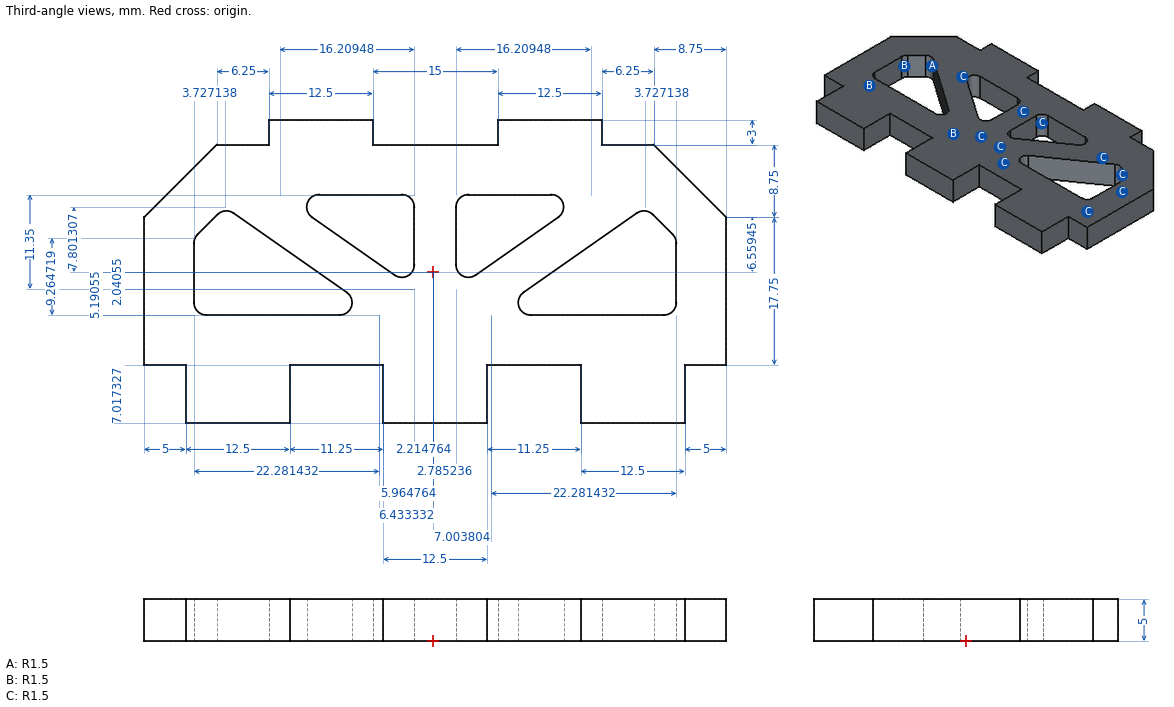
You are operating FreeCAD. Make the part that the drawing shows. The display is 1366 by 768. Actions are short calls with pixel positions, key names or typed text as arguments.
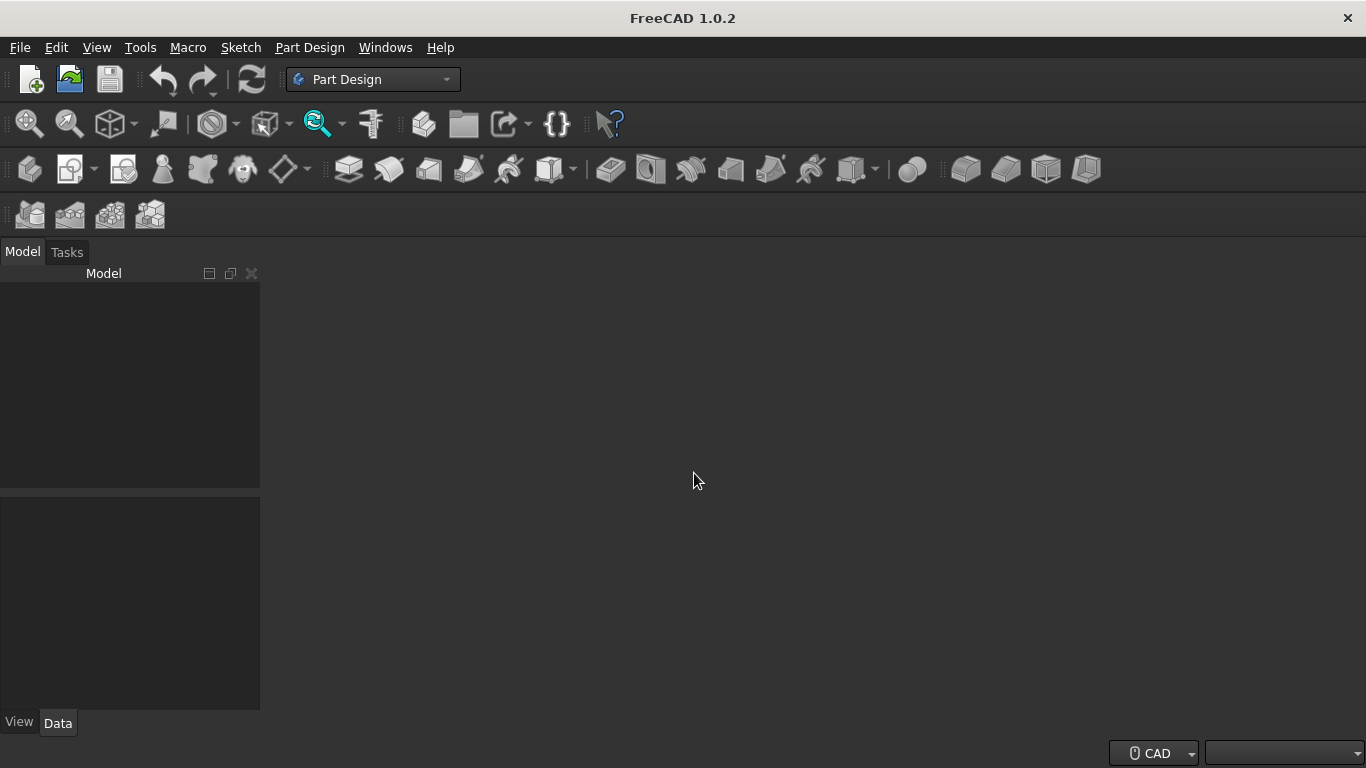
key(ctrl+n)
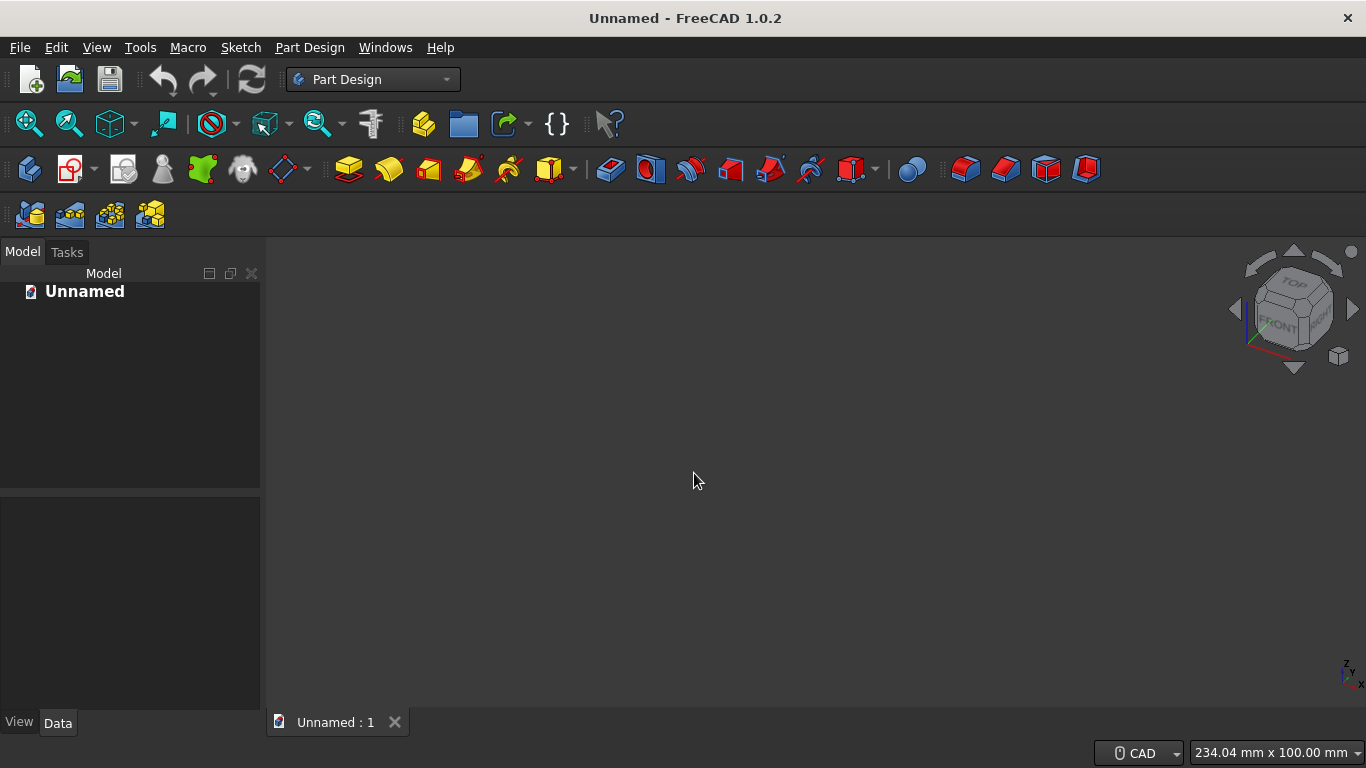
click(70, 170)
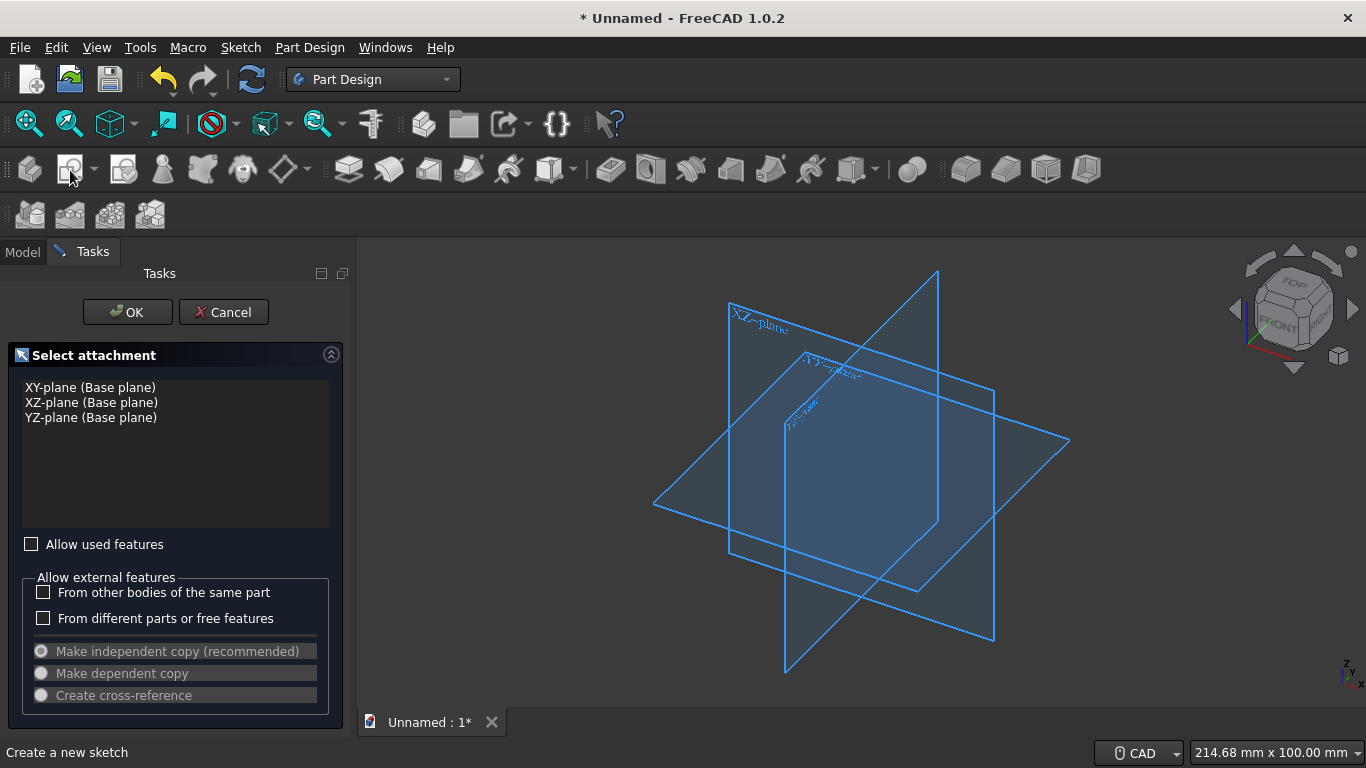
click(82, 388)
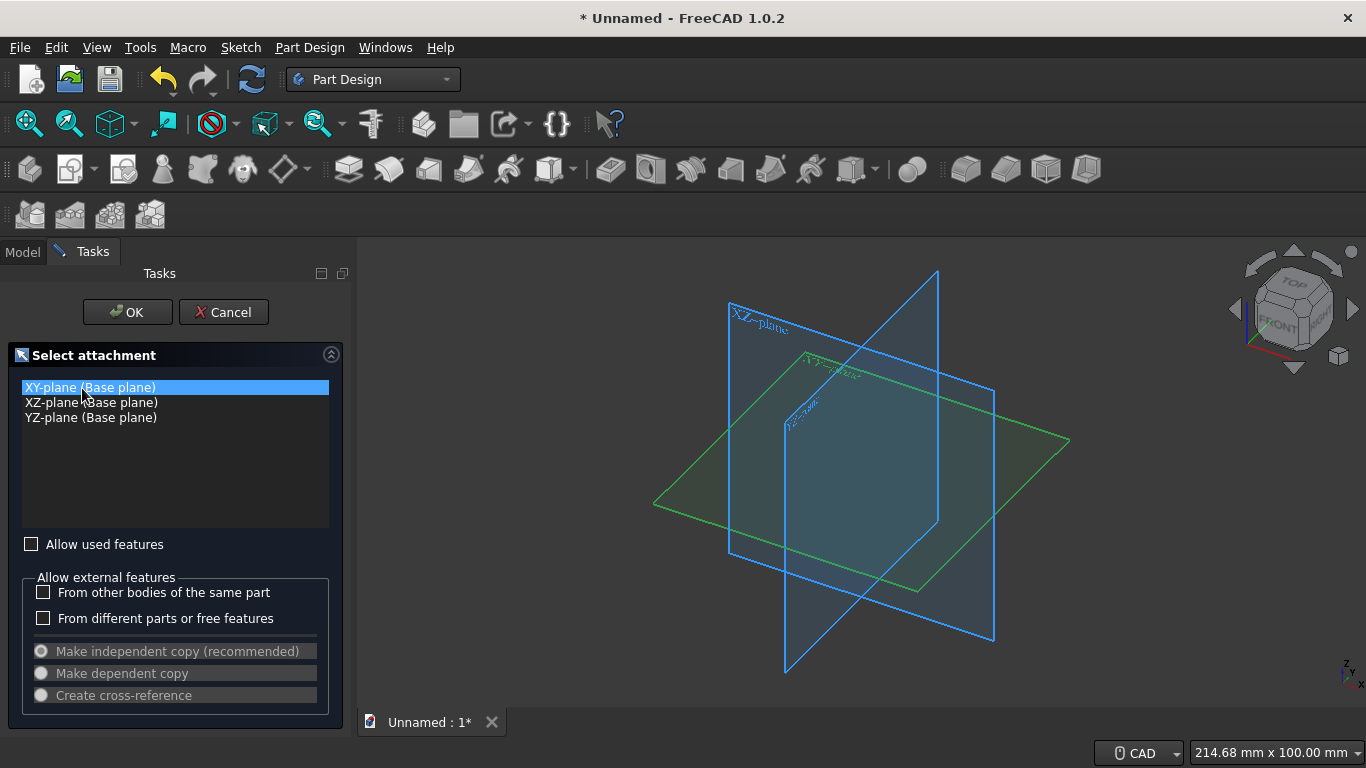
click(128, 312)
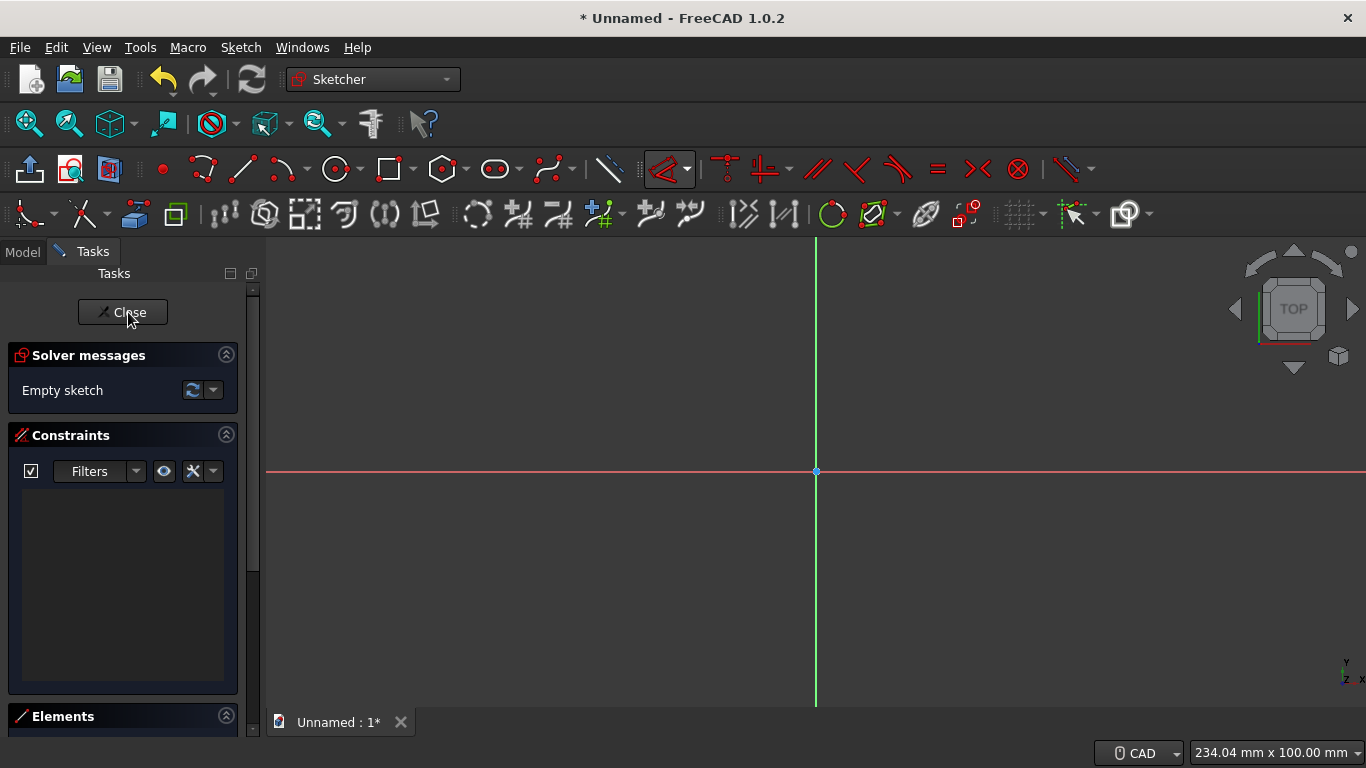
scroll(902, 471, up, 3)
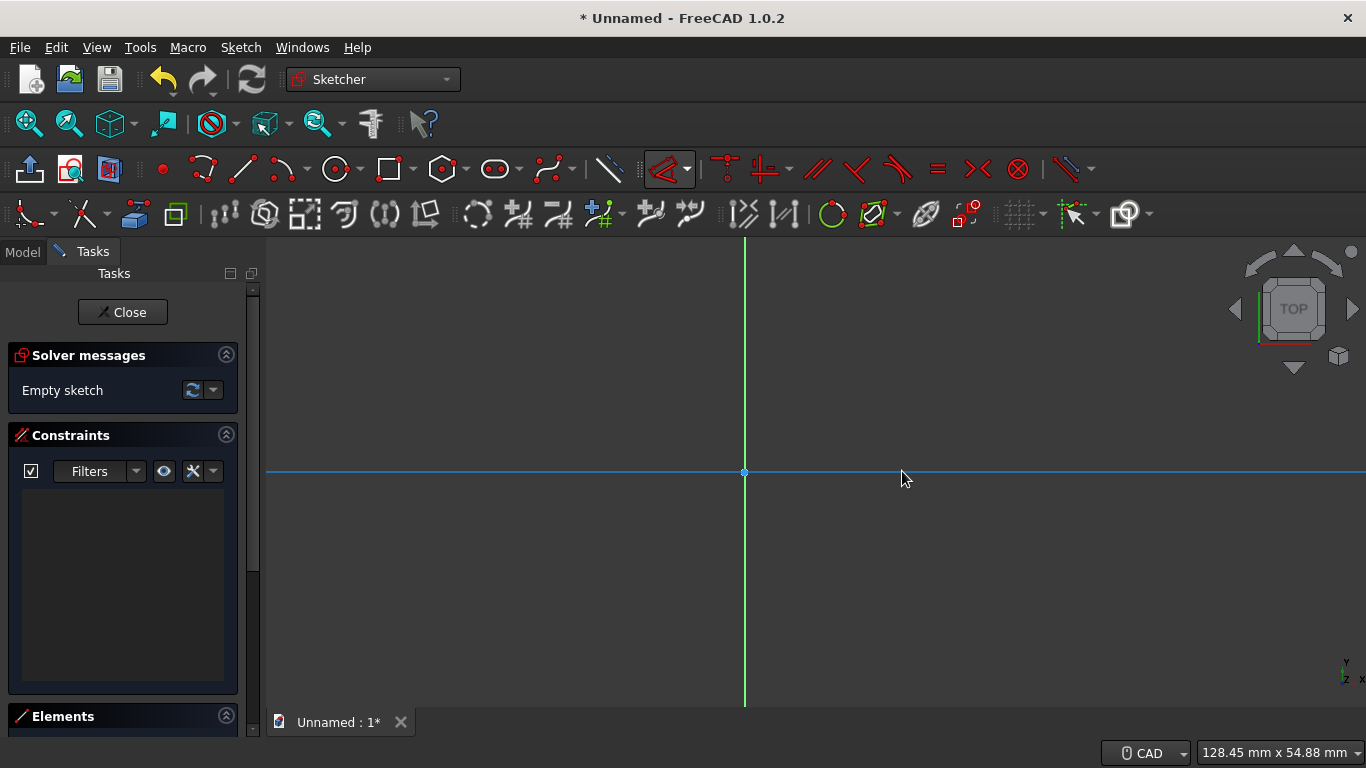
key(g)
key(m)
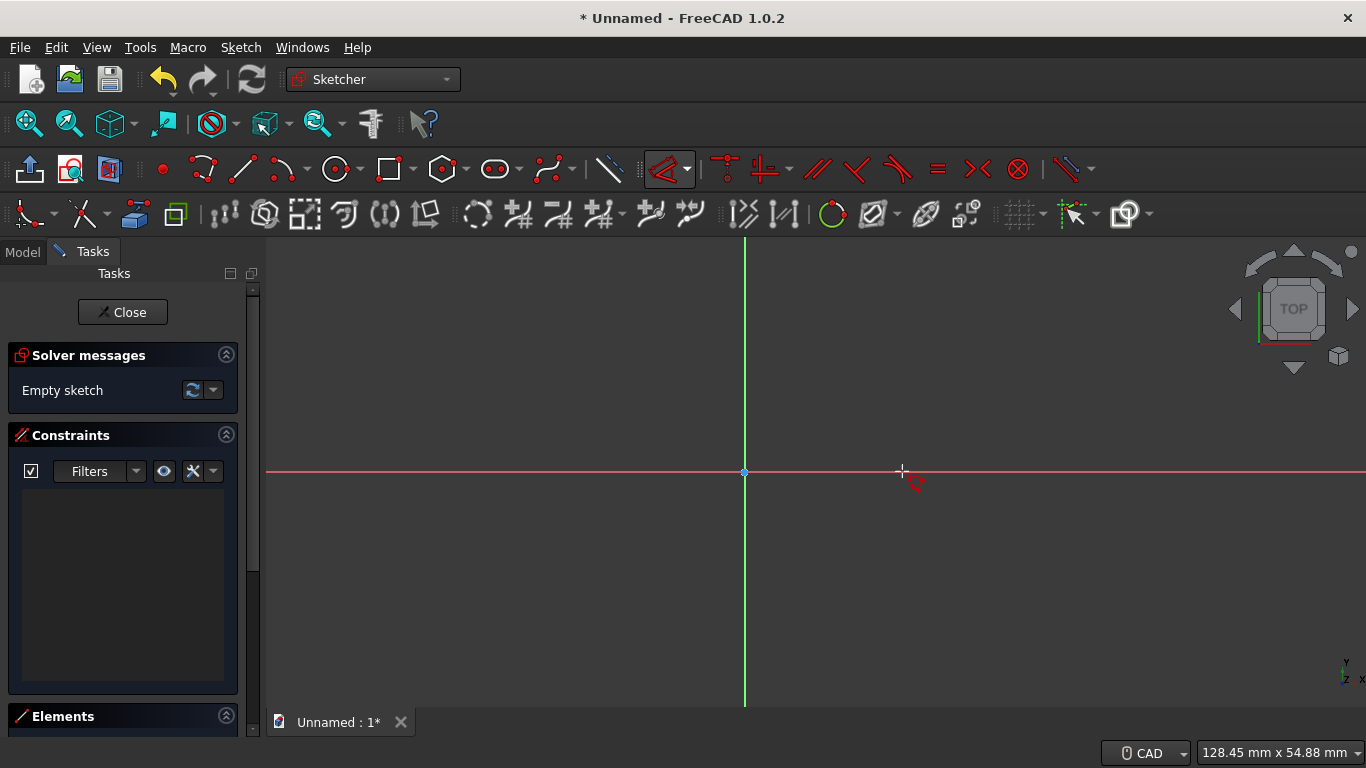
click(694, 568)
click(694, 628)
click(801, 628)
click(801, 568)
click(897, 568)
click(897, 628)
click(1004, 628)
click(1004, 568)
click(1047, 568)
click(1047, 416)
click(972, 341)
click(919, 341)
click(919, 316)
click(811, 316)
click(811, 341)
click(683, 341)
click(683, 316)
click(576, 316)
click(576, 341)
click(522, 341)
click(448, 416)
click(448, 568)
click(490, 568)
click(490, 628)
click(597, 628)
click(597, 568)
click(694, 569)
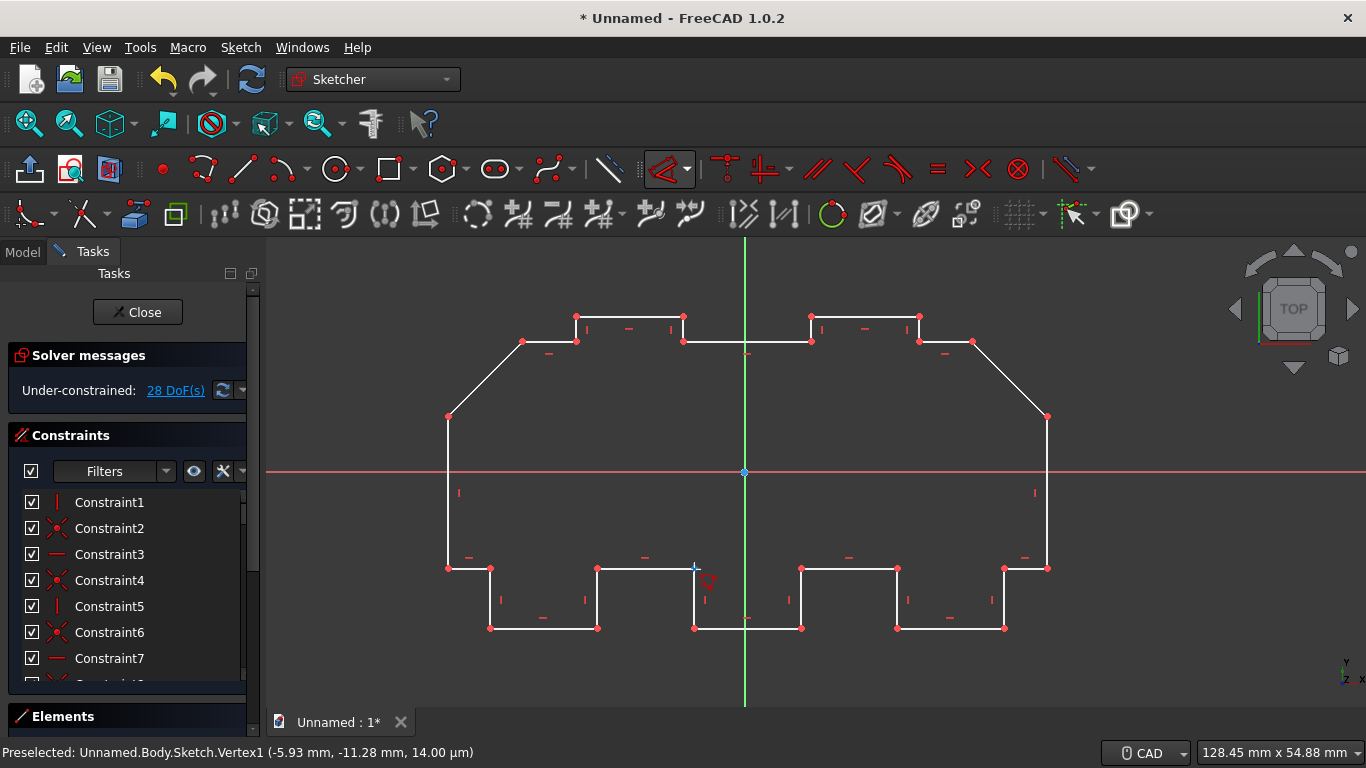
click(690, 517)
click(499, 517)
click(499, 438)
click(531, 406)
click(690, 518)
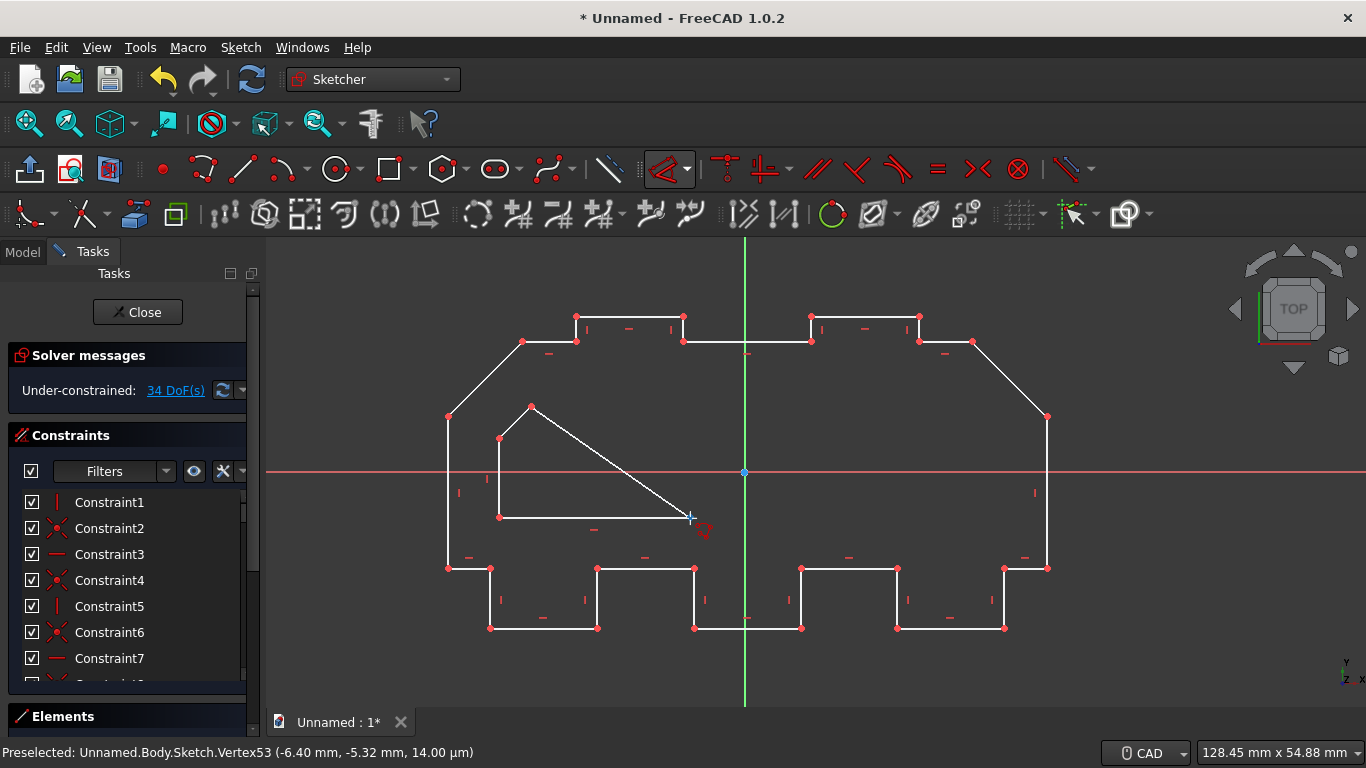
click(805, 517)
click(964, 406)
click(996, 438)
click(996, 517)
click(805, 518)